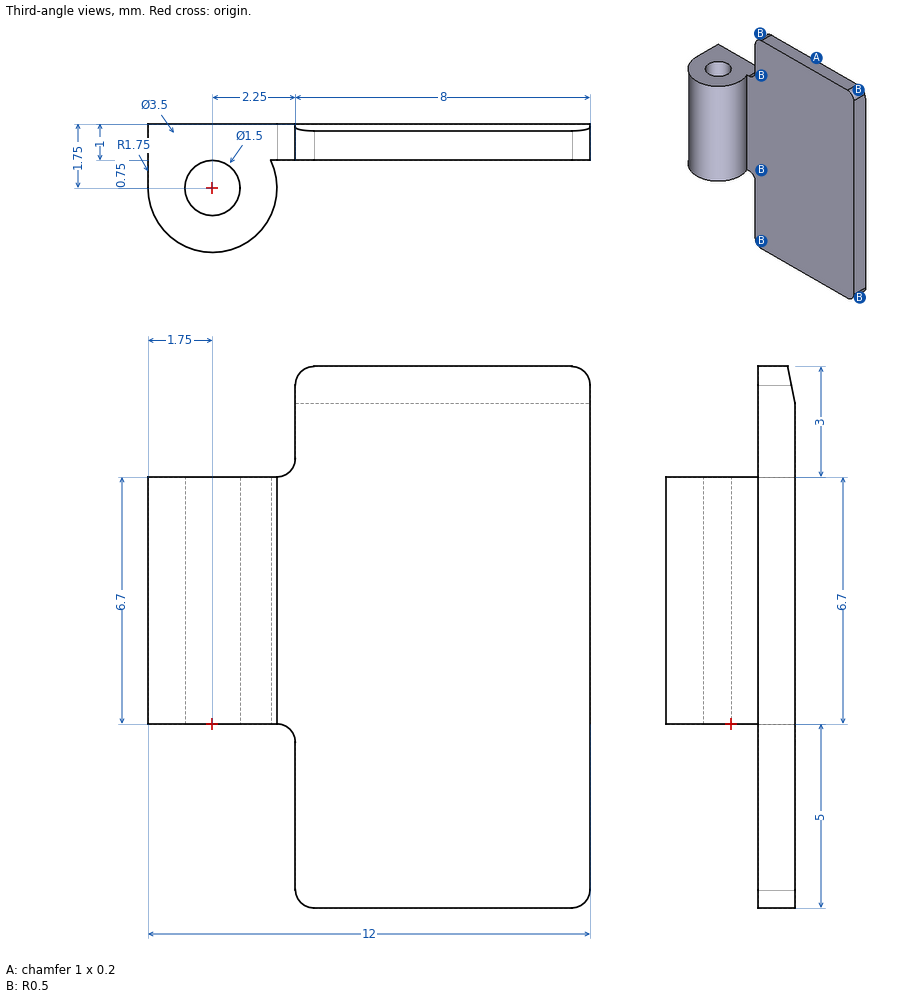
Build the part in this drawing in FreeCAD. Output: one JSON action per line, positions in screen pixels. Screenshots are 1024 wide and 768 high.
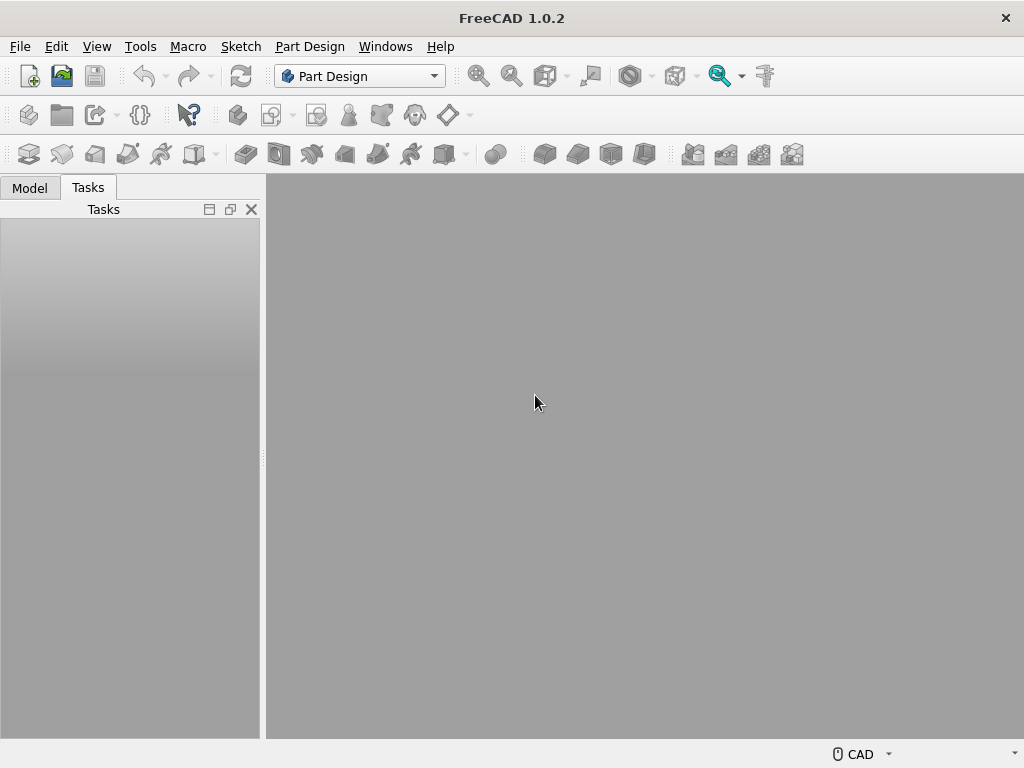
{"action": "left_click", "coordinate": [29, 76]}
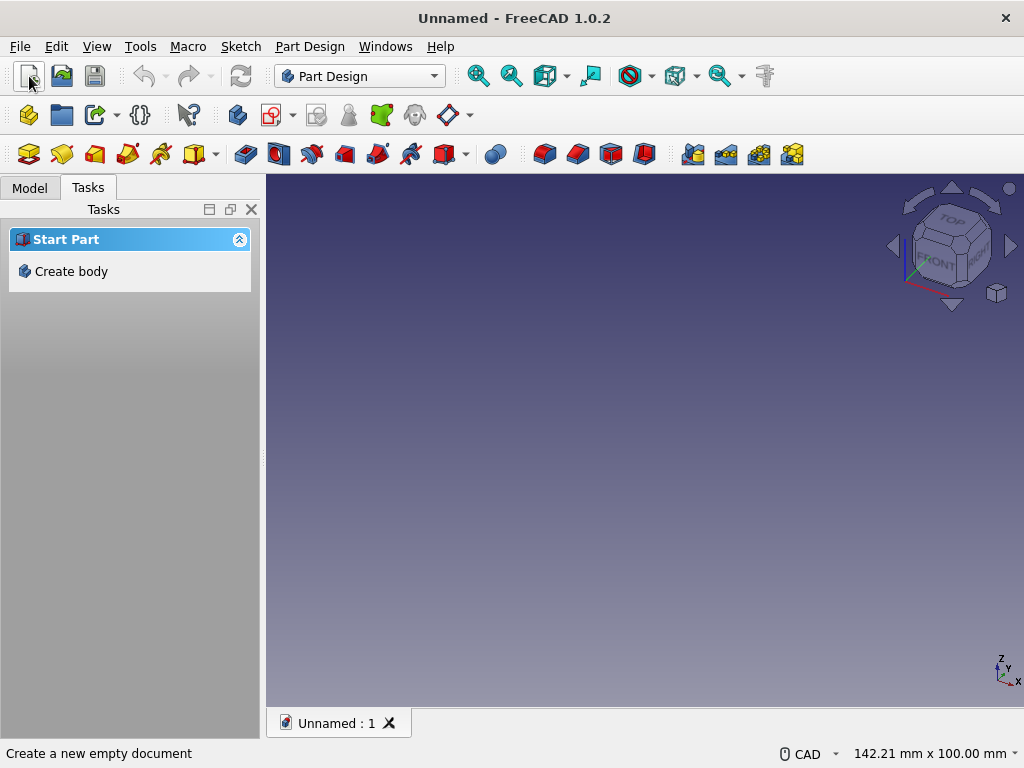
{"action": "left_click", "coordinate": [270, 116]}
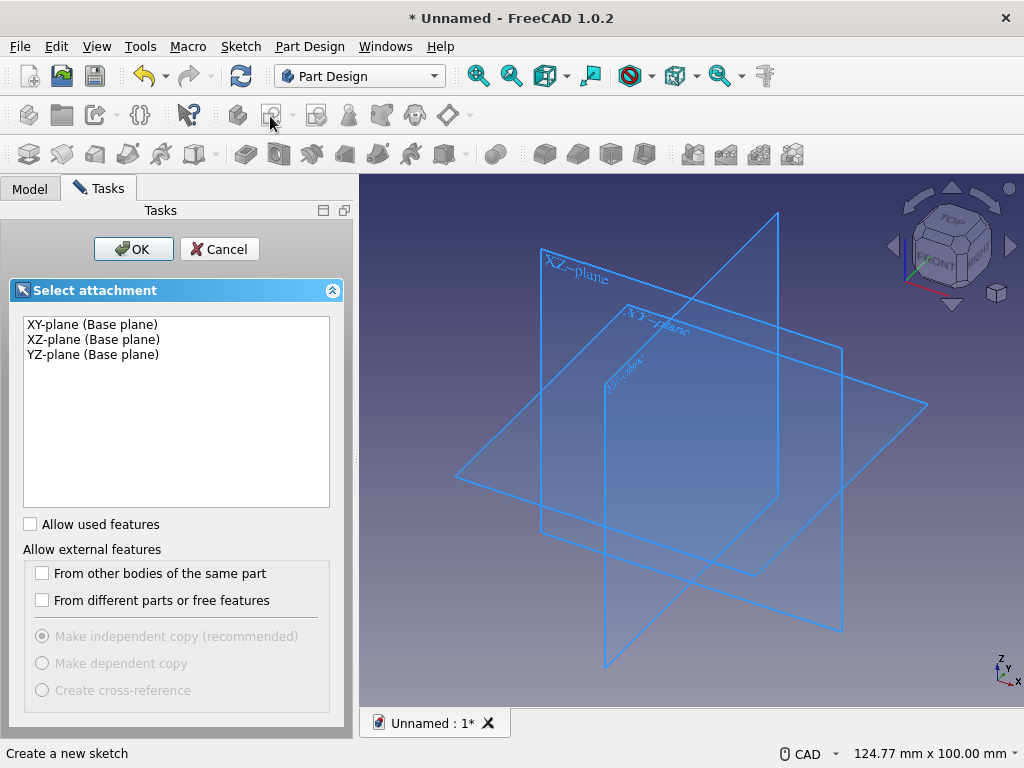
{"action": "left_click", "coordinate": [84, 324]}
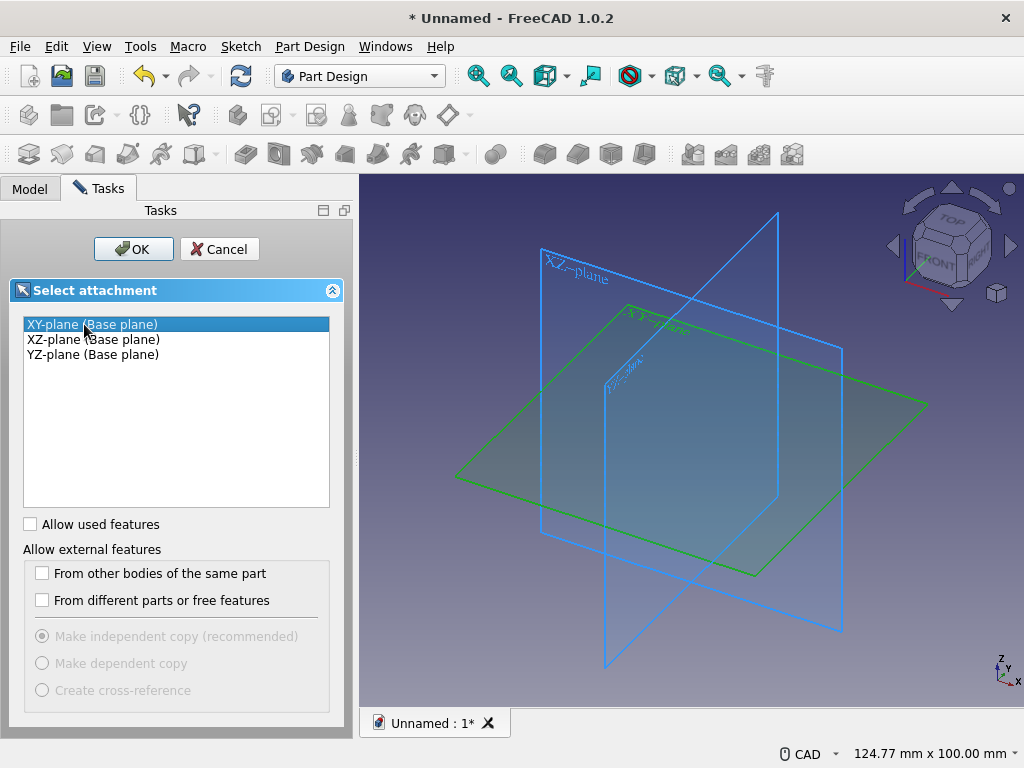
{"action": "left_click", "coordinate": [134, 249]}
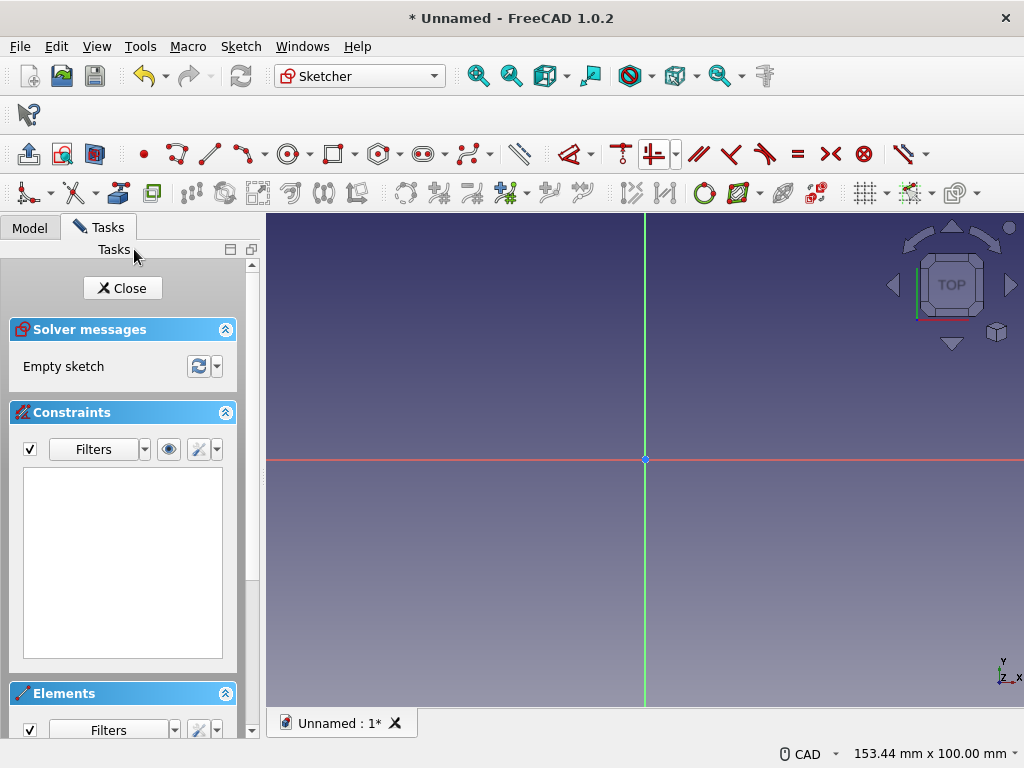
{"action": "scroll", "coordinate": [649, 460], "scroll_direction": "up", "scroll_amount": 14}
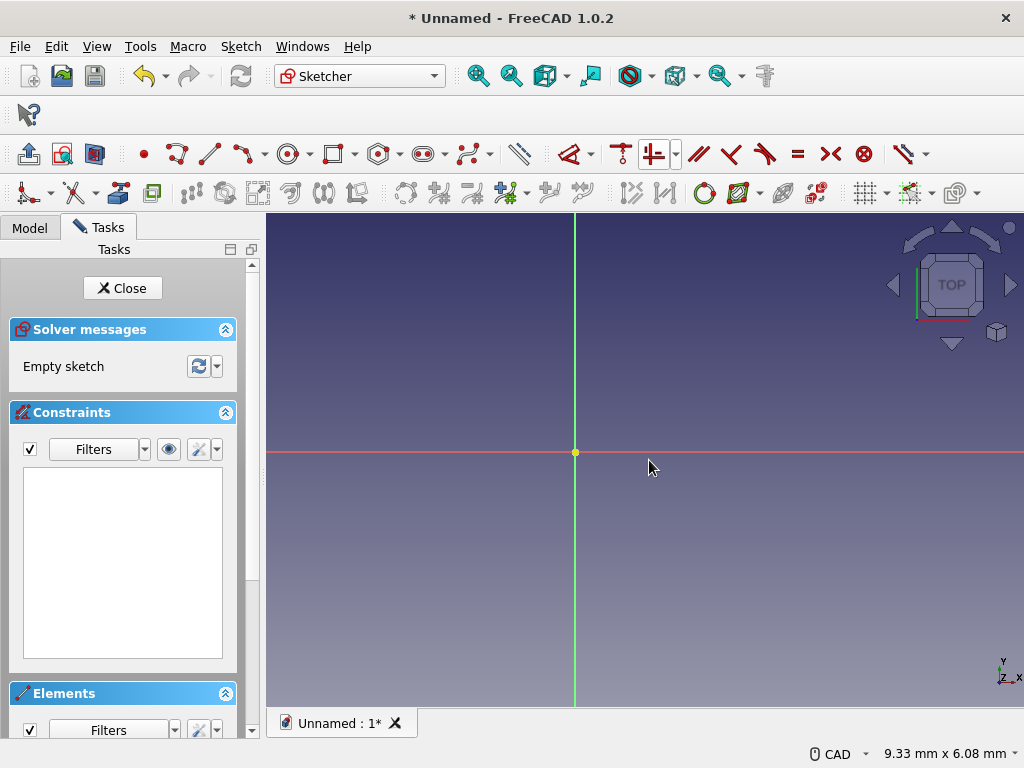
{"action": "left_click", "coordinate": [288, 154]}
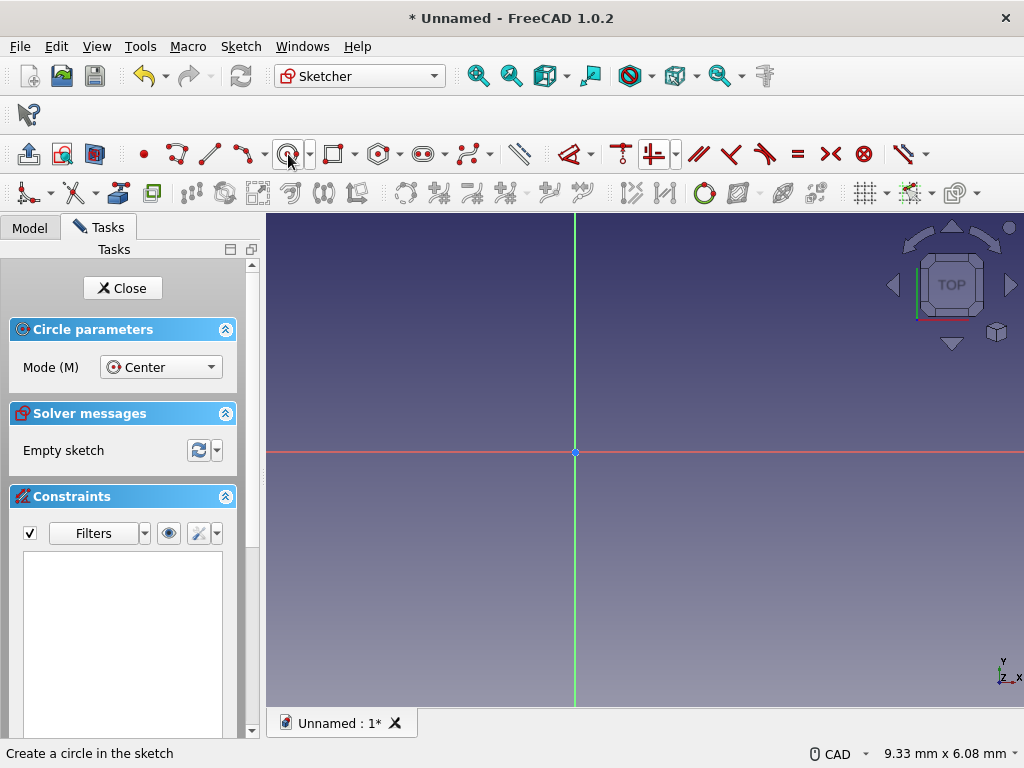
{"action": "left_click", "coordinate": [575, 452]}
{"action": "left_click", "coordinate": [676, 352]}
{"action": "key", "text": "Escape"}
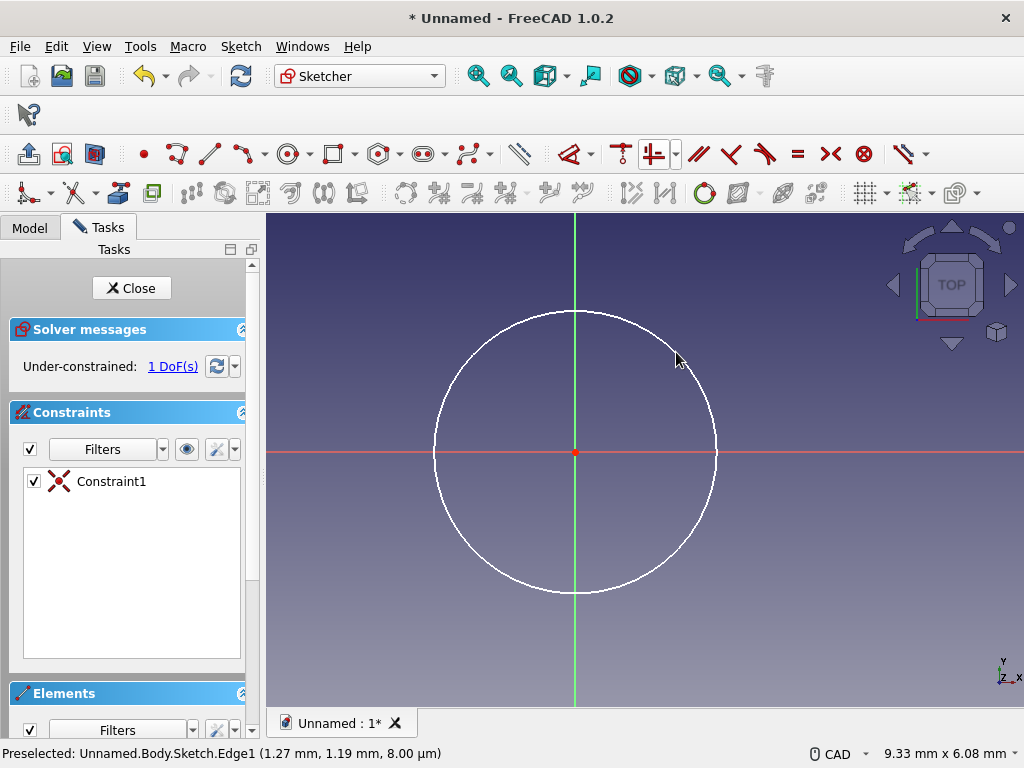
{"action": "left_click", "coordinate": [675, 352]}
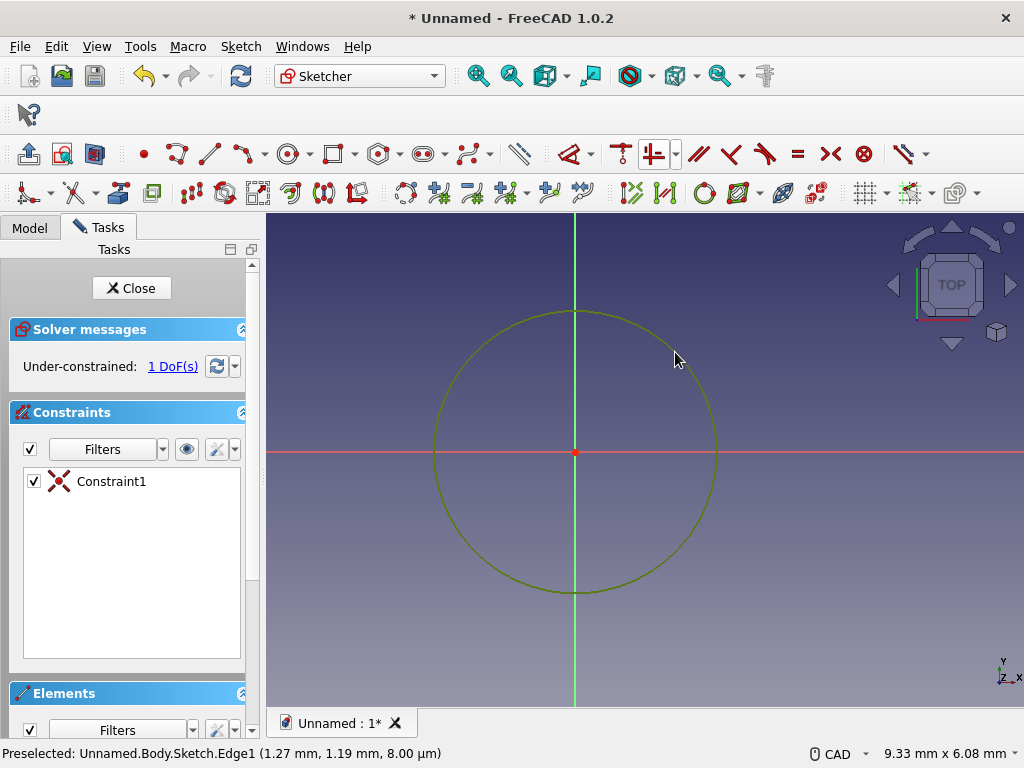
{"action": "key", "text": "k o"}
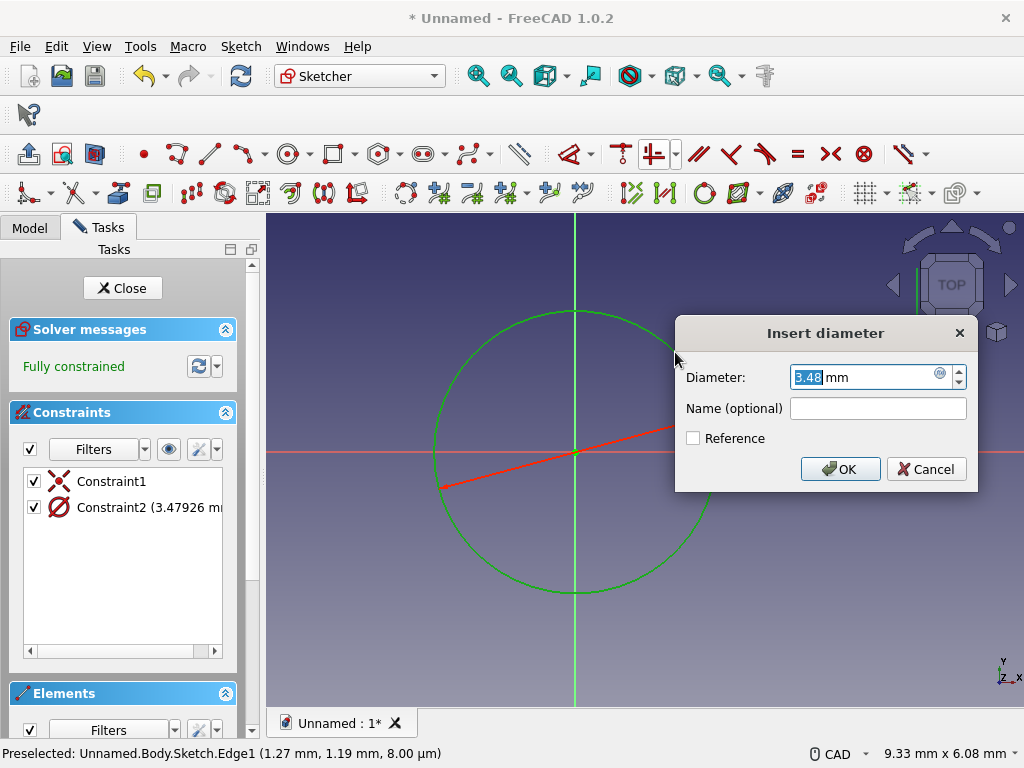
{"action": "type", "text": "3.5"}
{"action": "key", "text": "Return"}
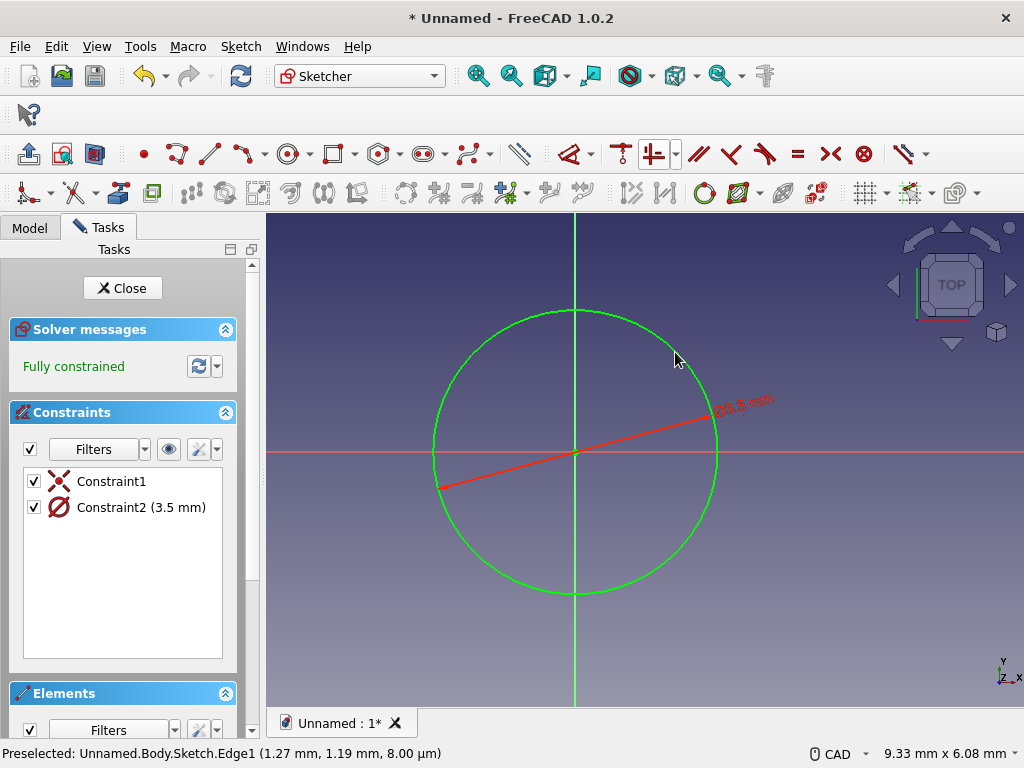
{"action": "left_click", "coordinate": [123, 288]}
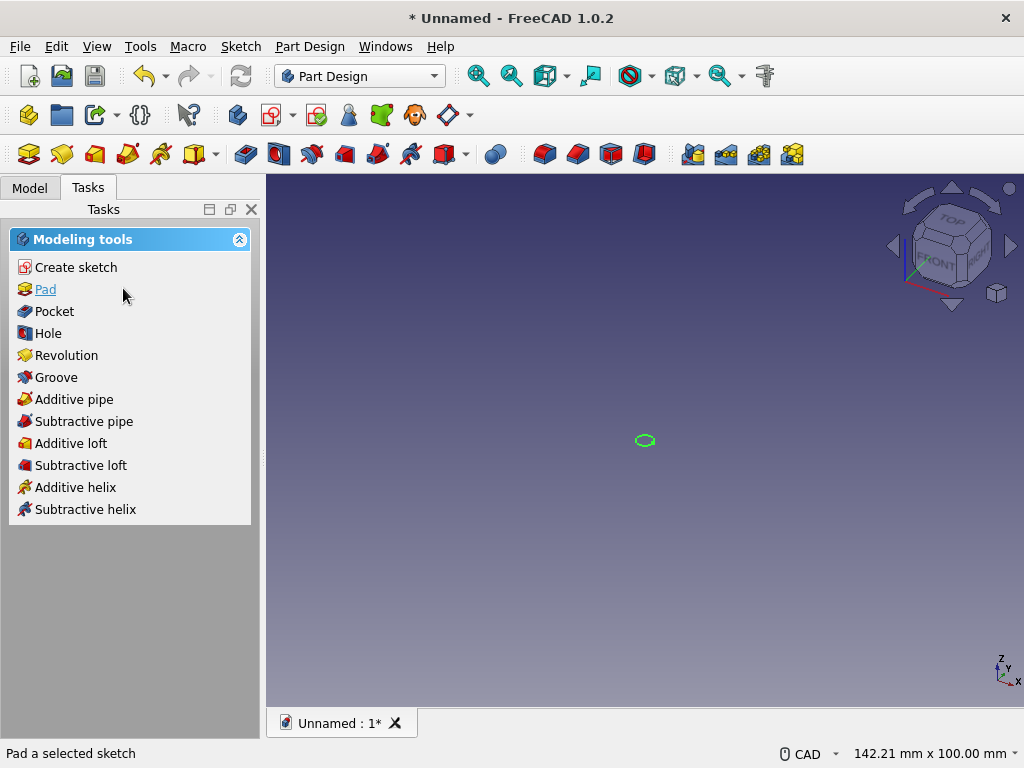
{"action": "left_click", "coordinate": [29, 154]}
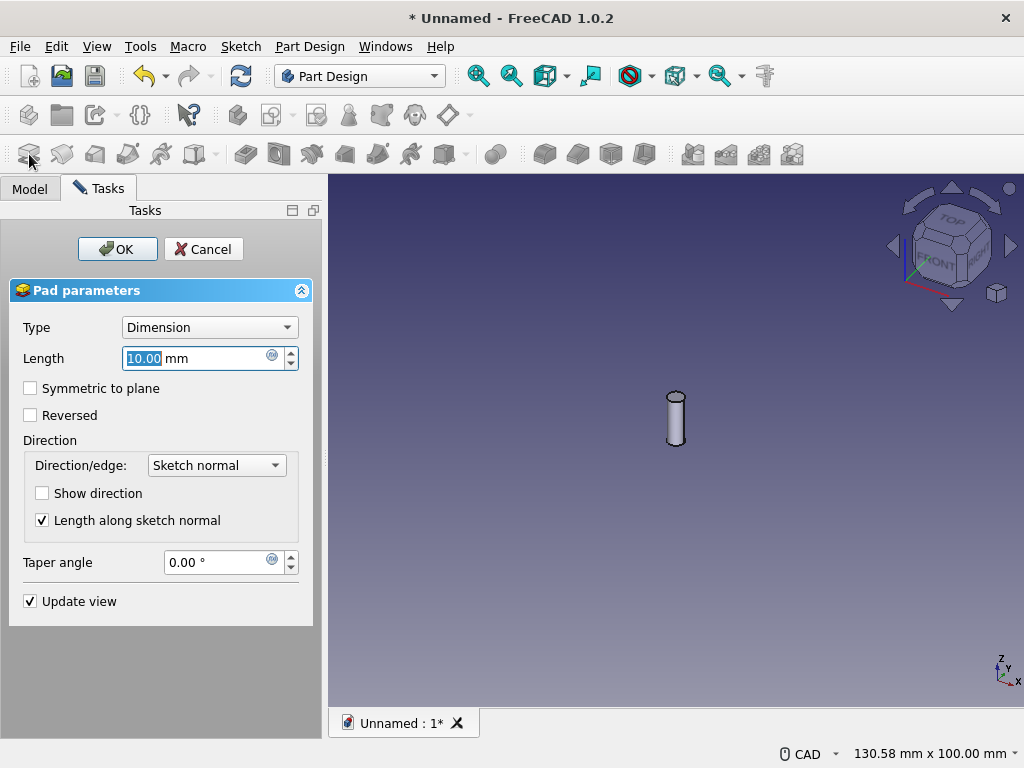
{"action": "type", "text": "6.7"}
{"action": "key", "text": "Tab"}